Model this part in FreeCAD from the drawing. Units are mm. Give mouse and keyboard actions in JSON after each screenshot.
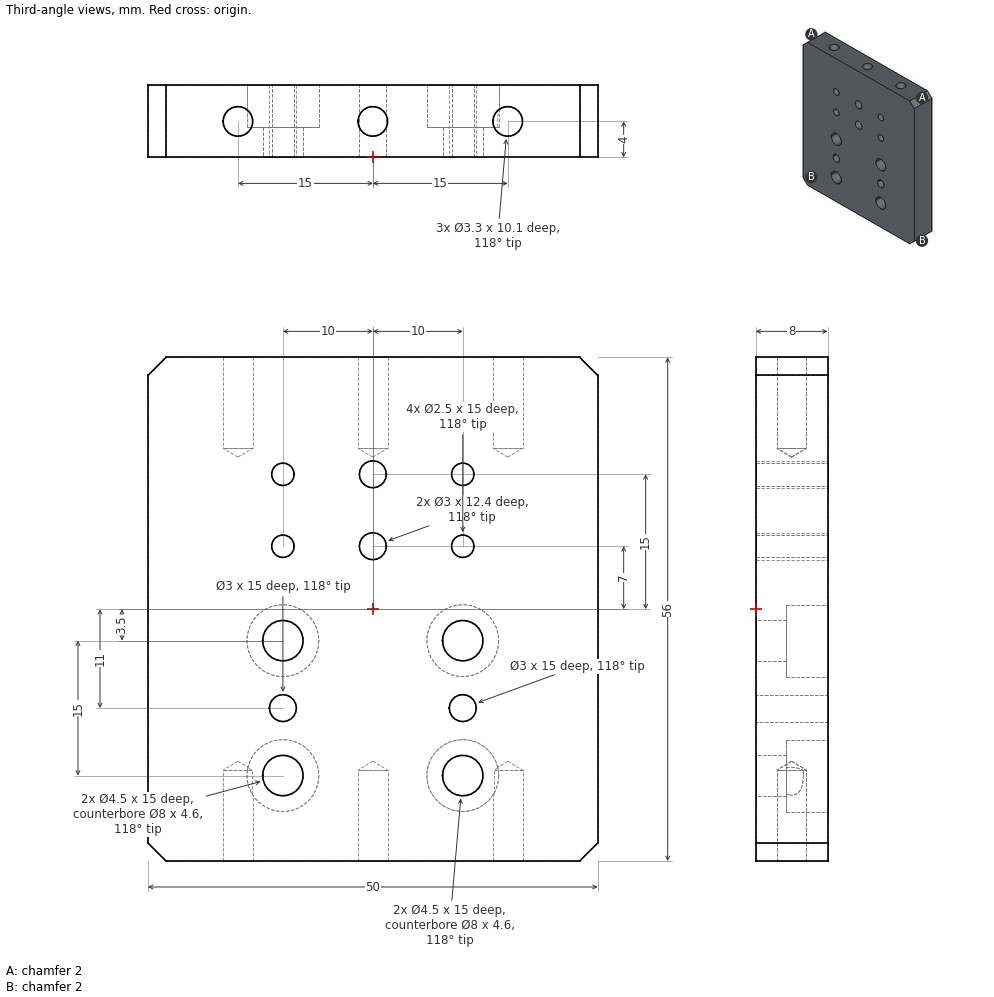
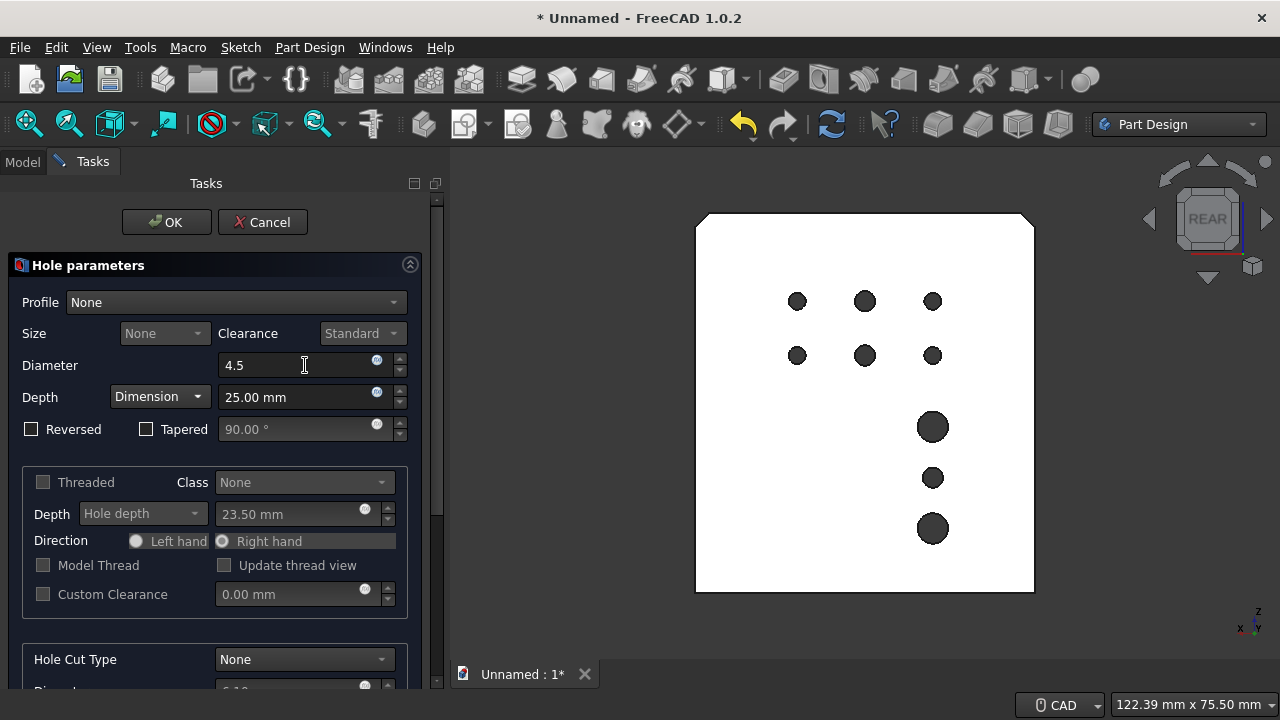
{"action": "triple_click", "coordinate": [305, 397]}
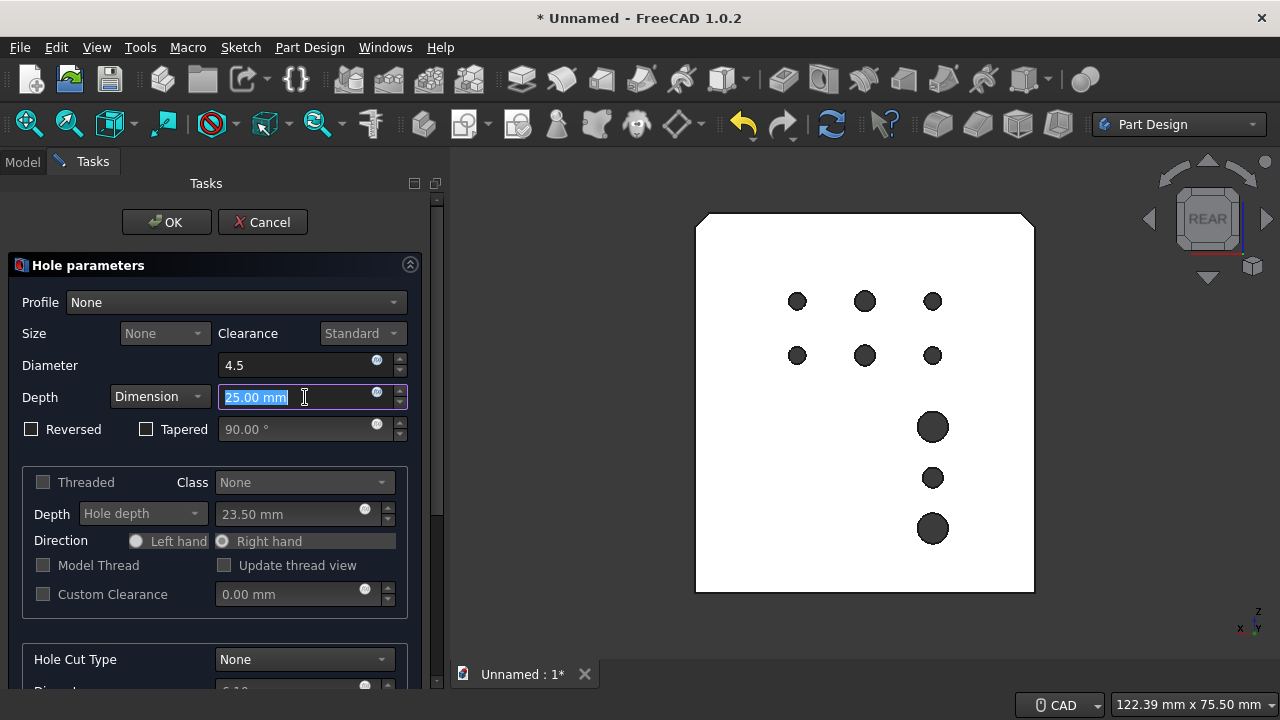
{"action": "type", "text": "15"}
{"action": "key", "text": "Tab"}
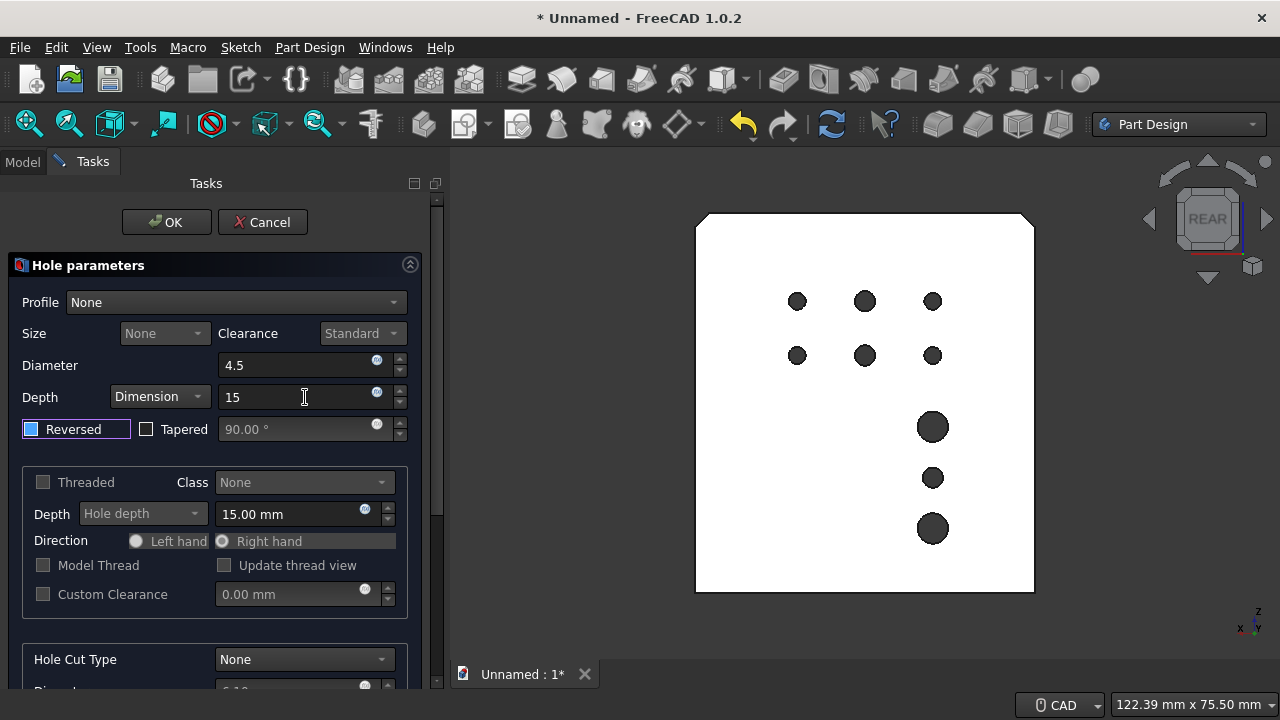
{"action": "left_click", "coordinate": [306, 660]}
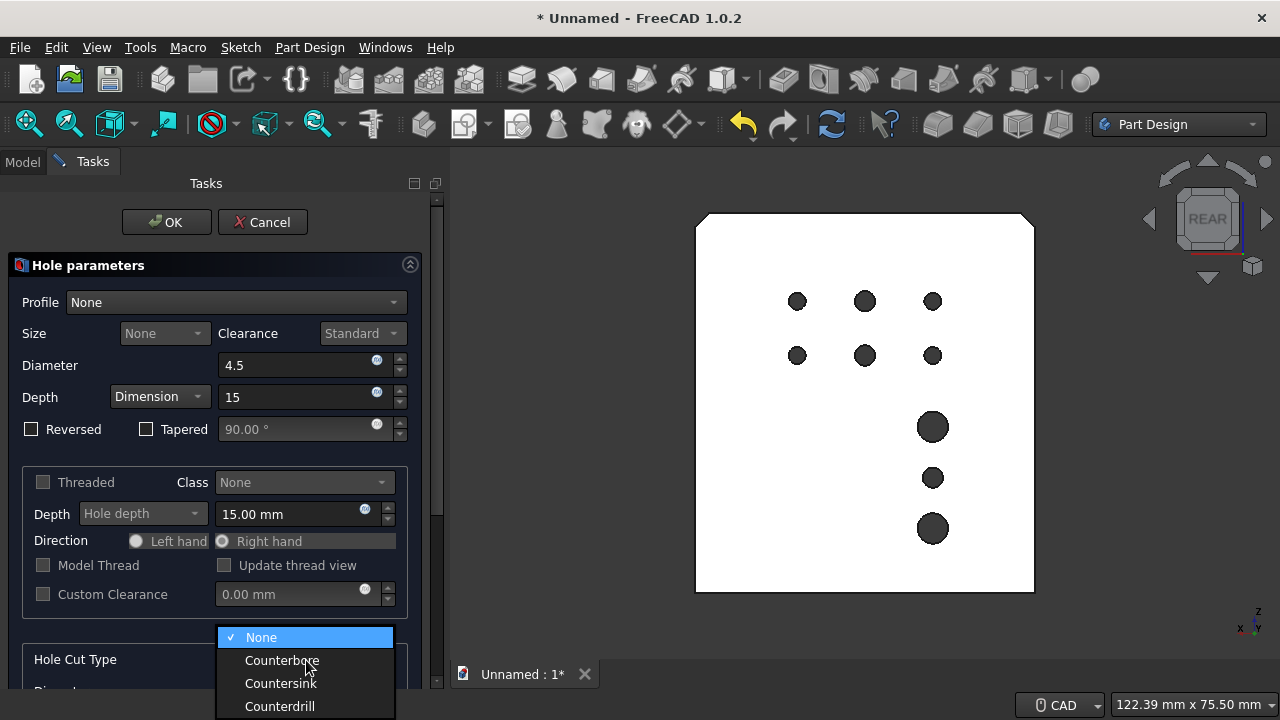
{"action": "left_click", "coordinate": [304, 660]}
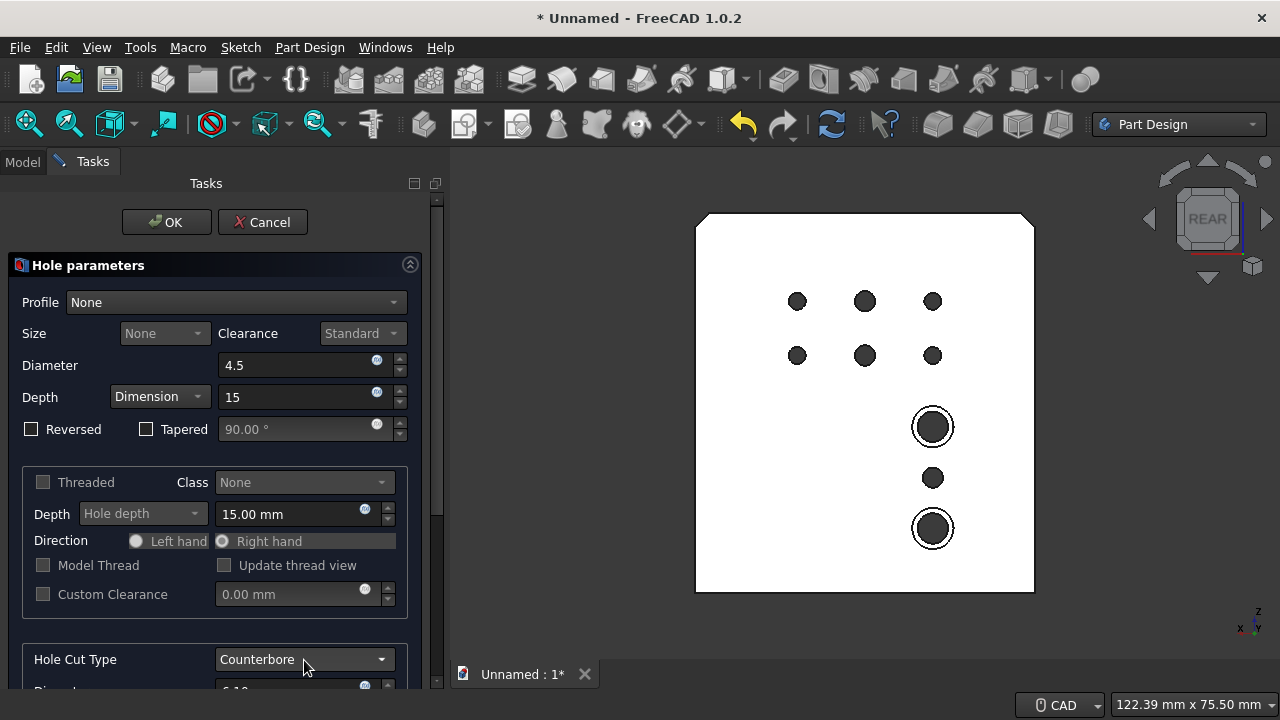
{"action": "scroll", "coordinate": [437, 440], "scroll_direction": "down", "scroll_amount": 2}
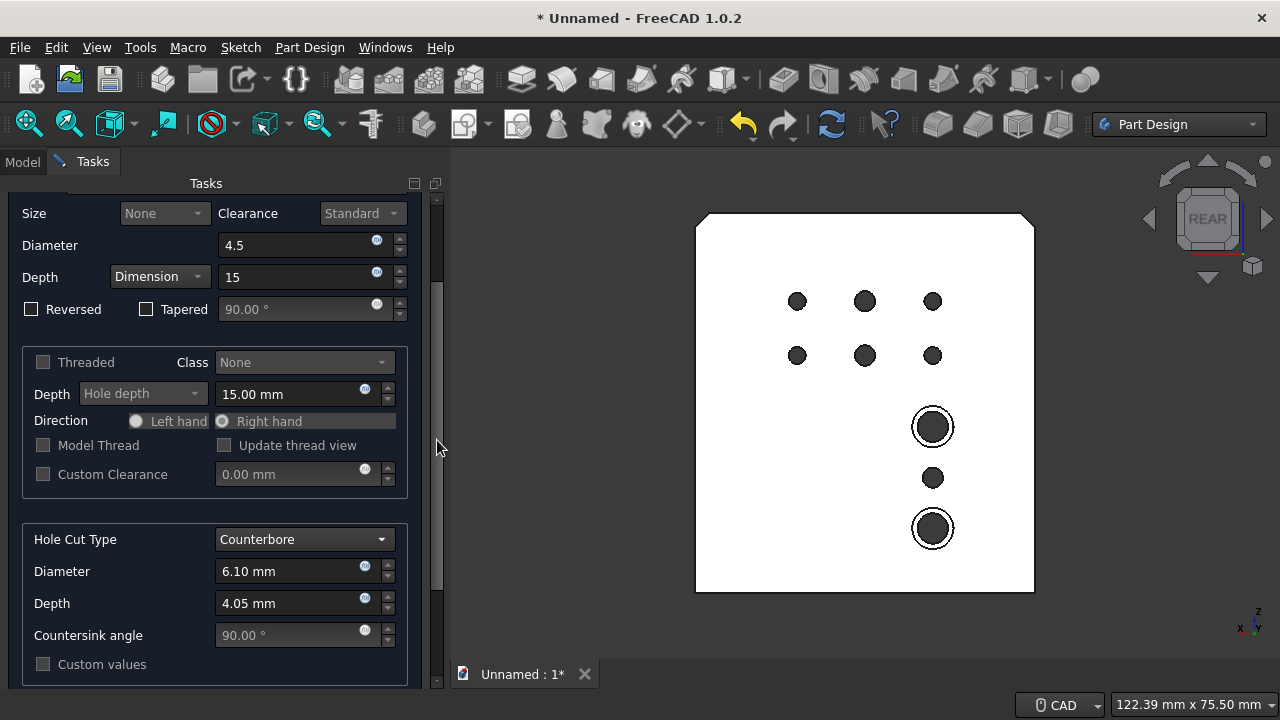
{"action": "triple_click", "coordinate": [298, 571]}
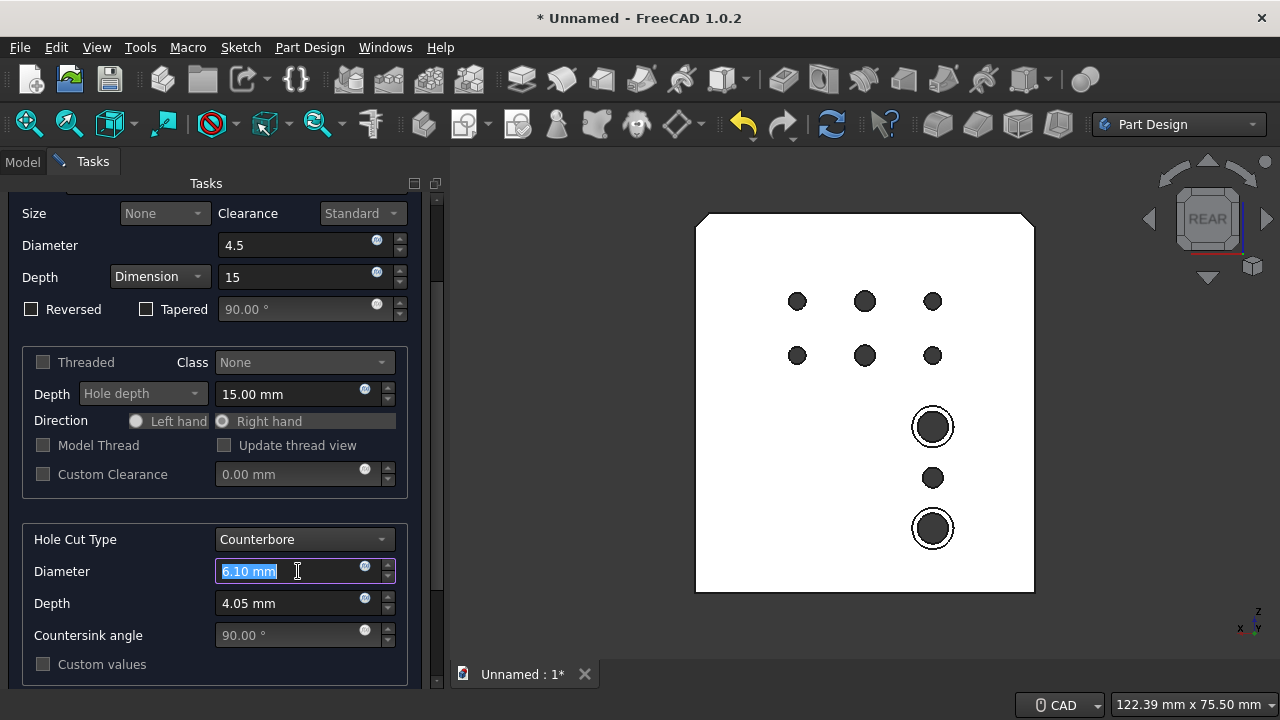
{"action": "type", "text": "8"}
{"action": "key", "text": "Tab"}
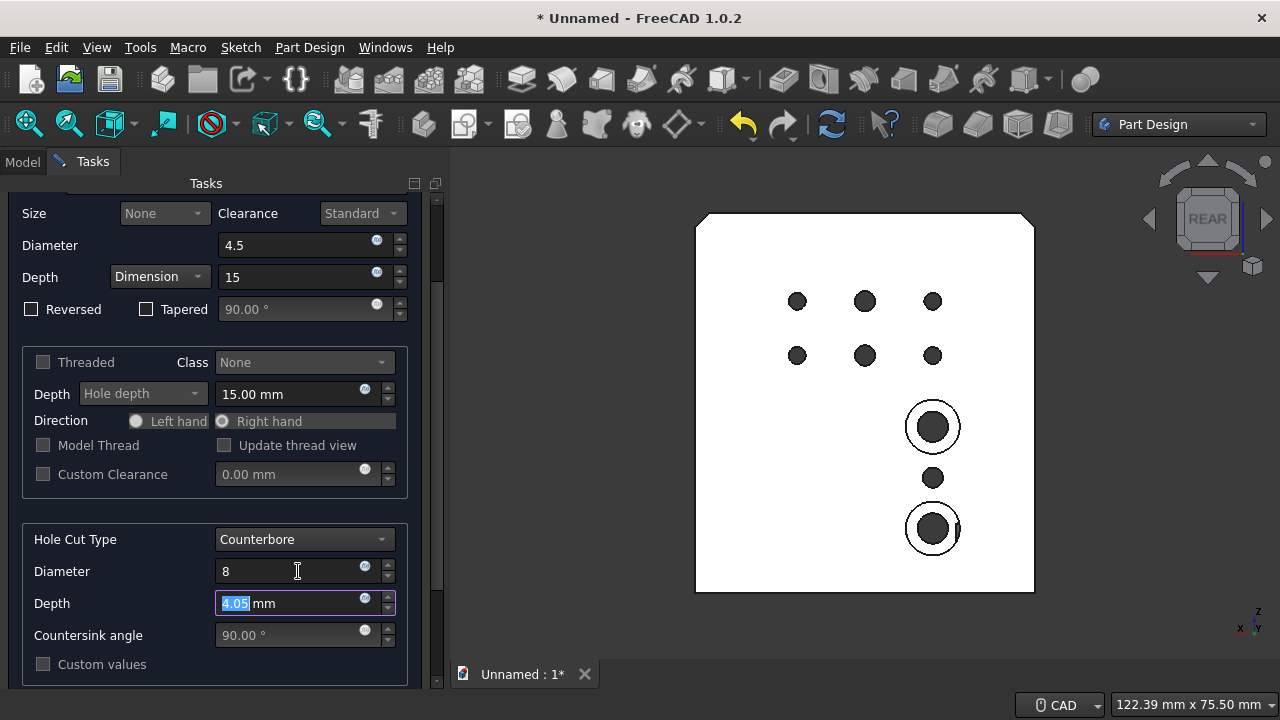
{"action": "type", "text": "4.6"}
{"action": "key", "text": "Tab"}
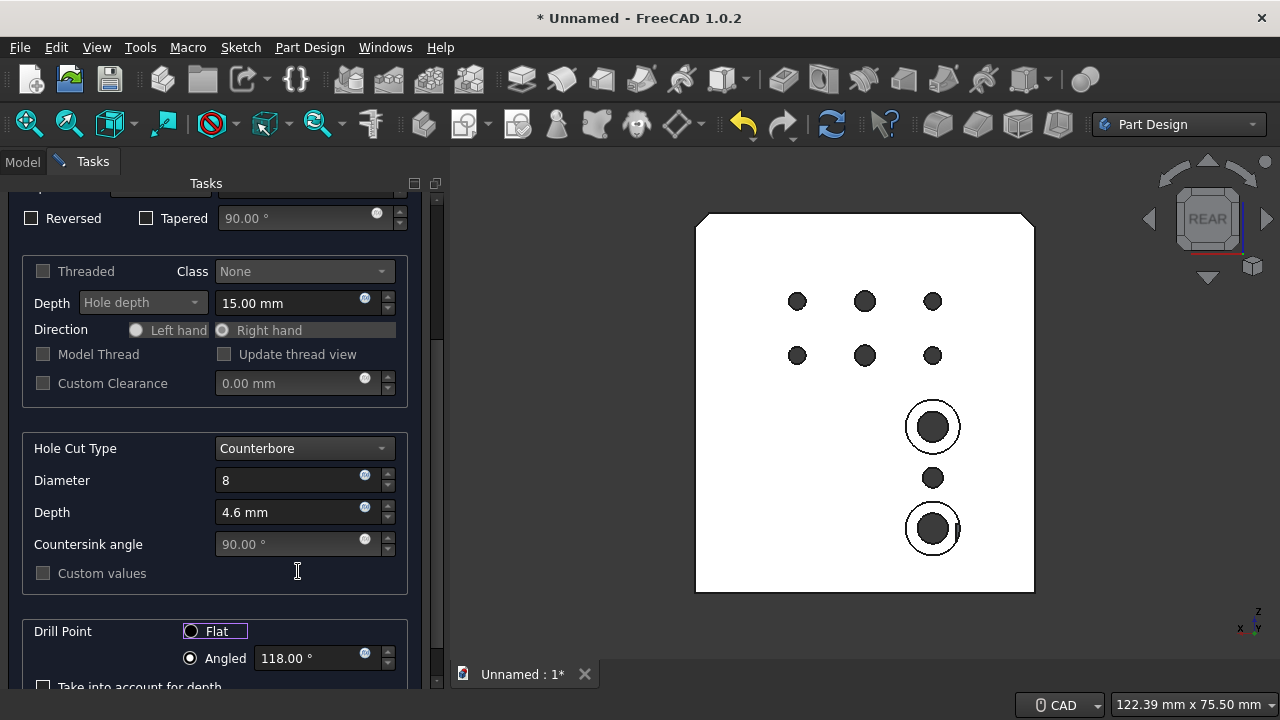
{"action": "scroll", "coordinate": [437, 440], "scroll_direction": "up", "scroll_amount": 5}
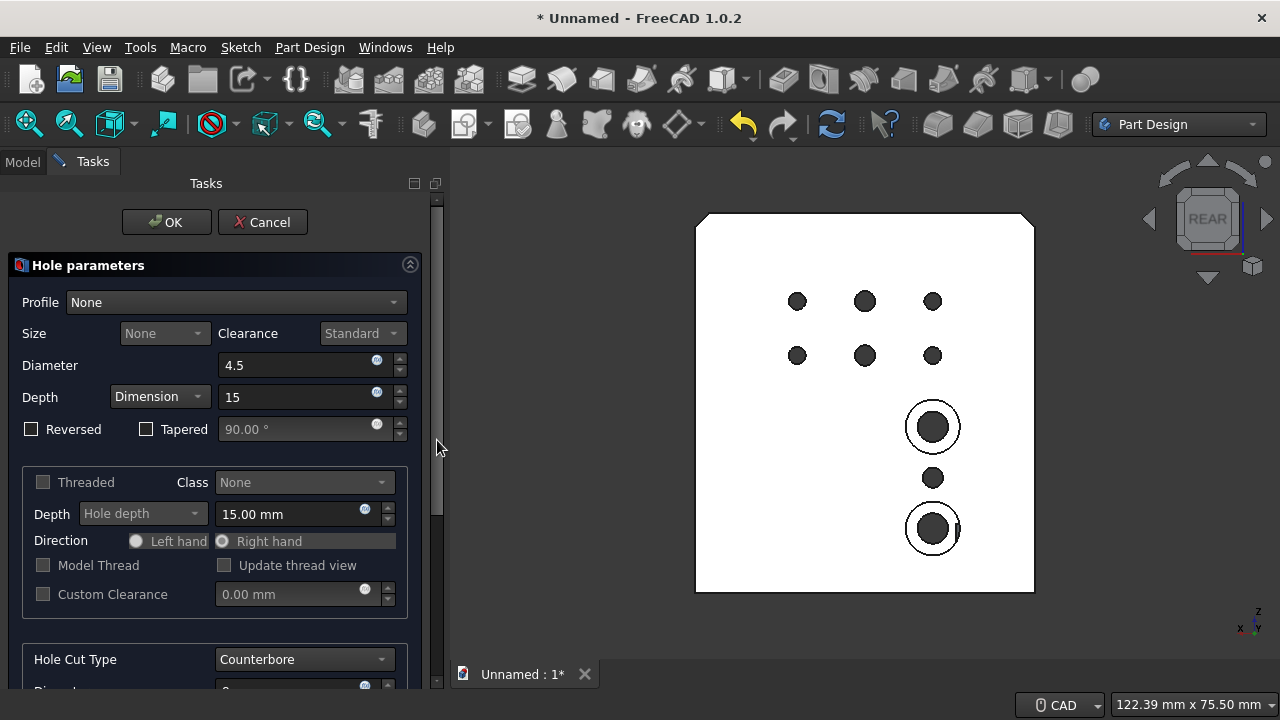
{"action": "left_click", "coordinate": [167, 222]}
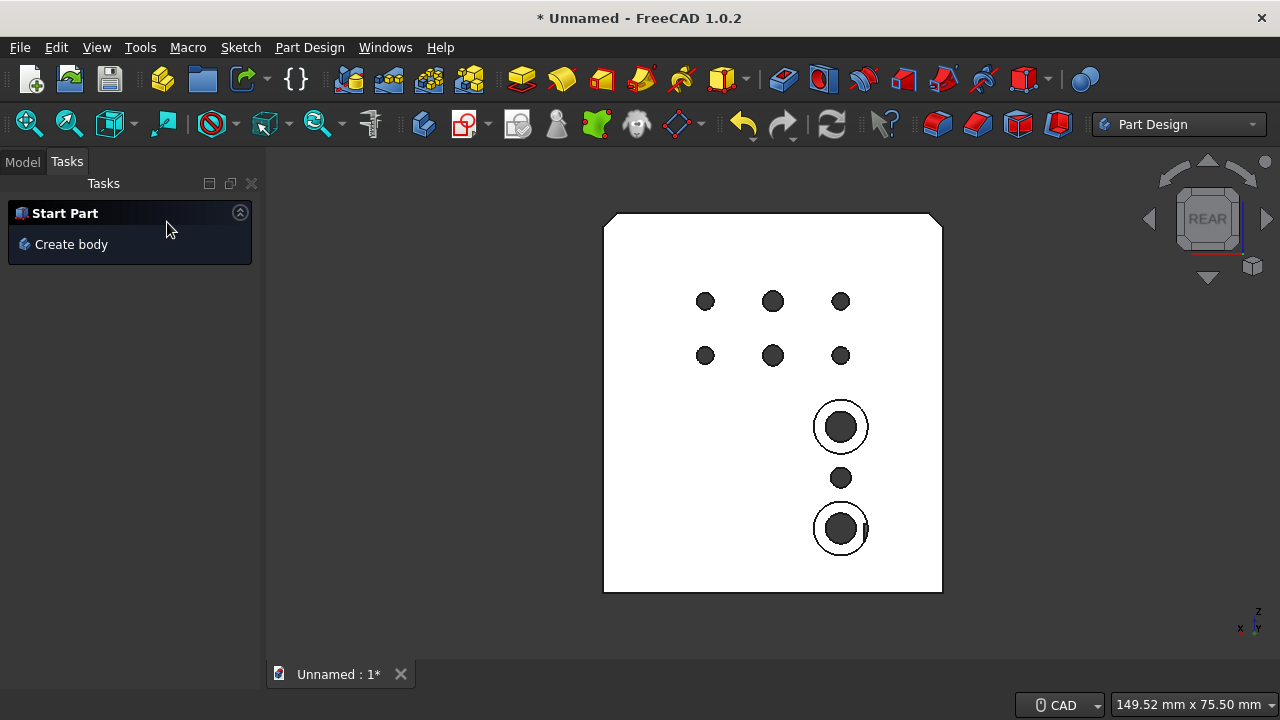
{"action": "left_click", "coordinate": [725, 456]}